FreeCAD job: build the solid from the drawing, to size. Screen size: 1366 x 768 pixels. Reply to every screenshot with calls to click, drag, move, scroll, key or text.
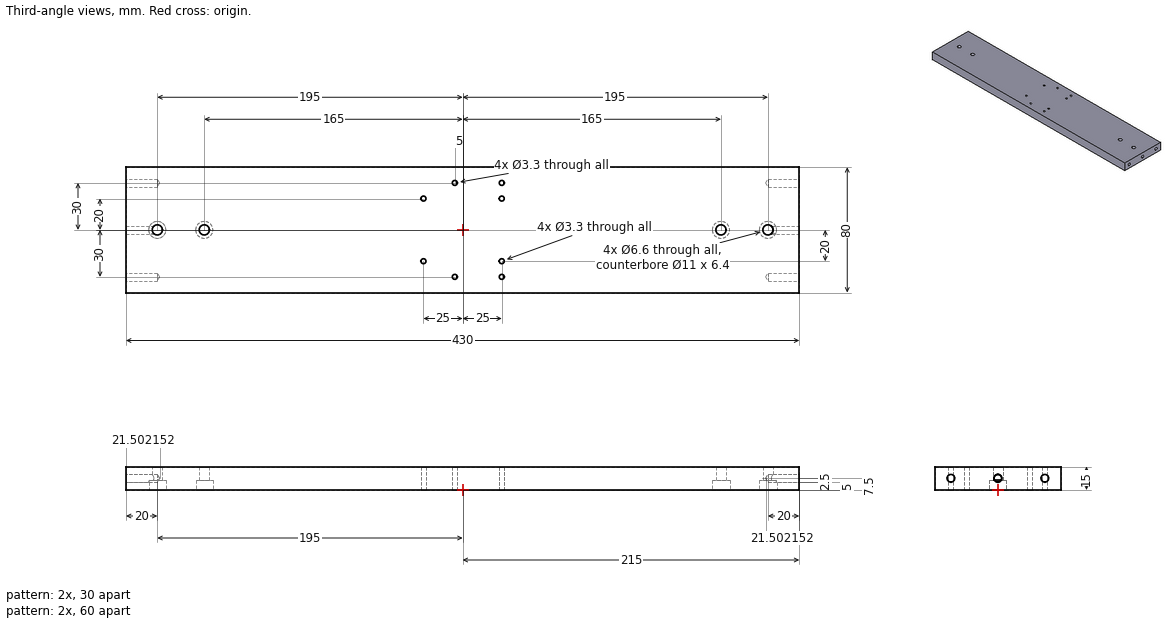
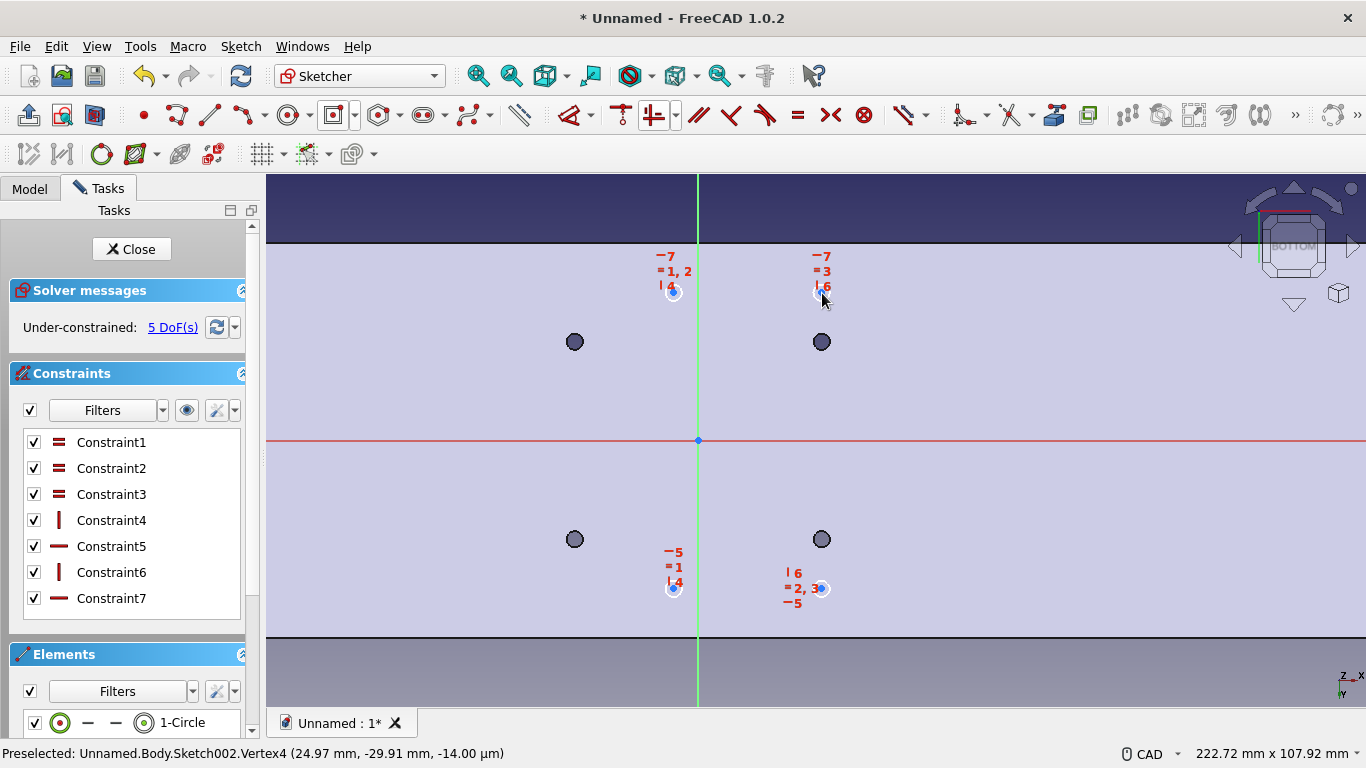
click(568, 116)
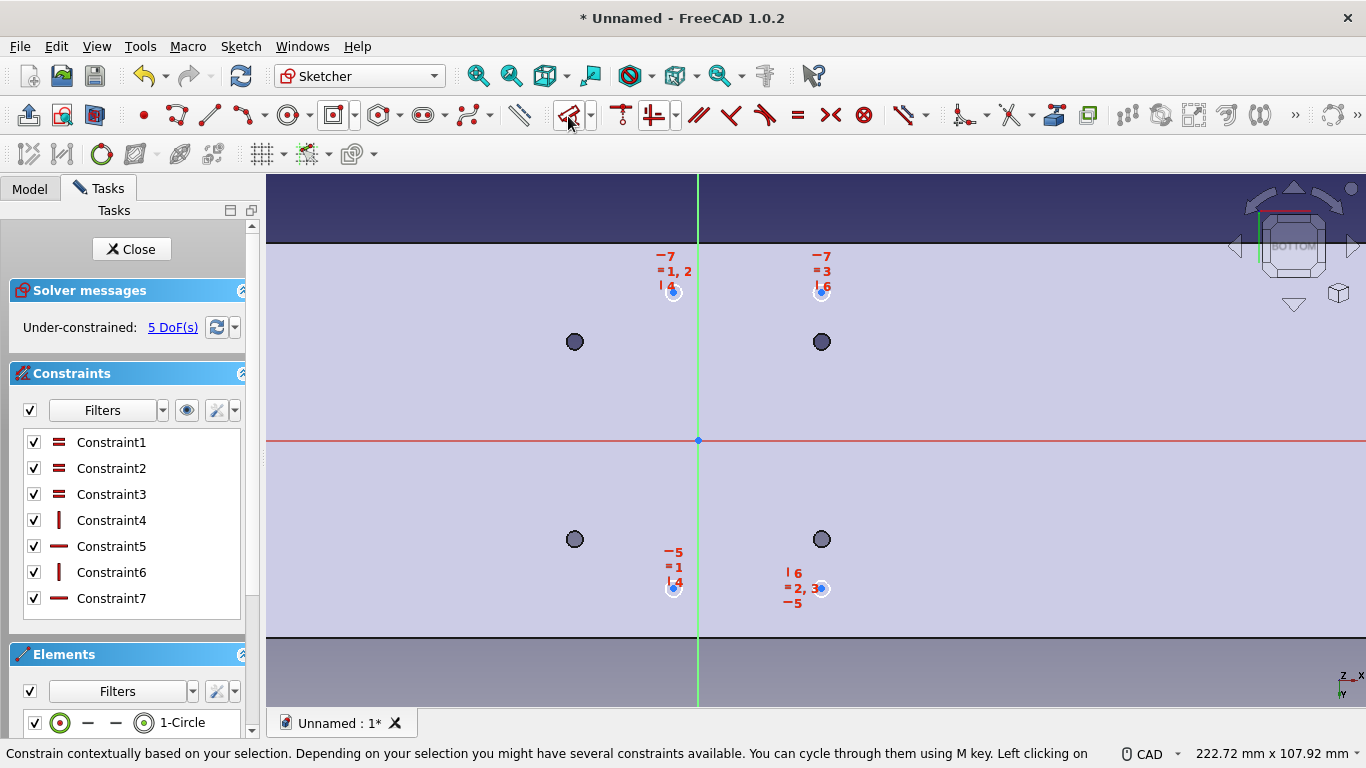
scroll(679, 583, up, 5)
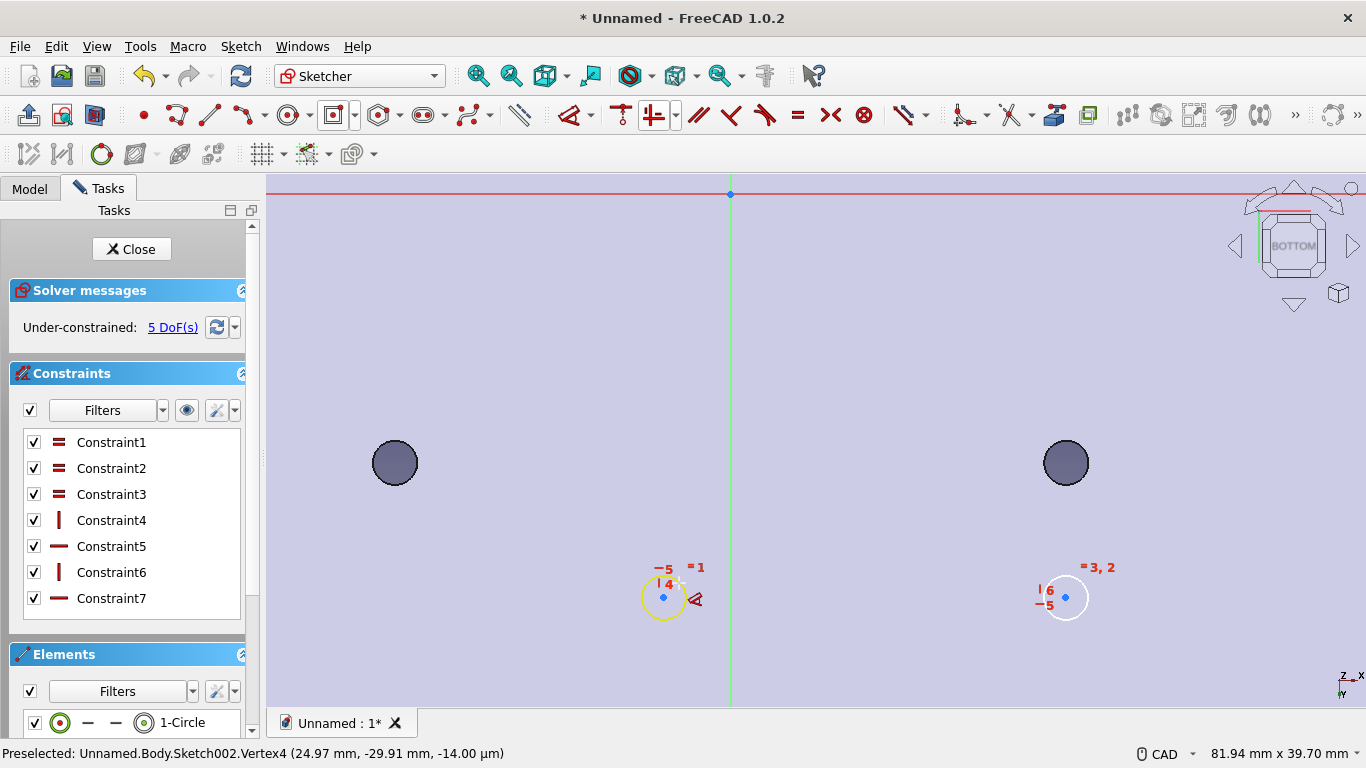
click(679, 582)
click(701, 559)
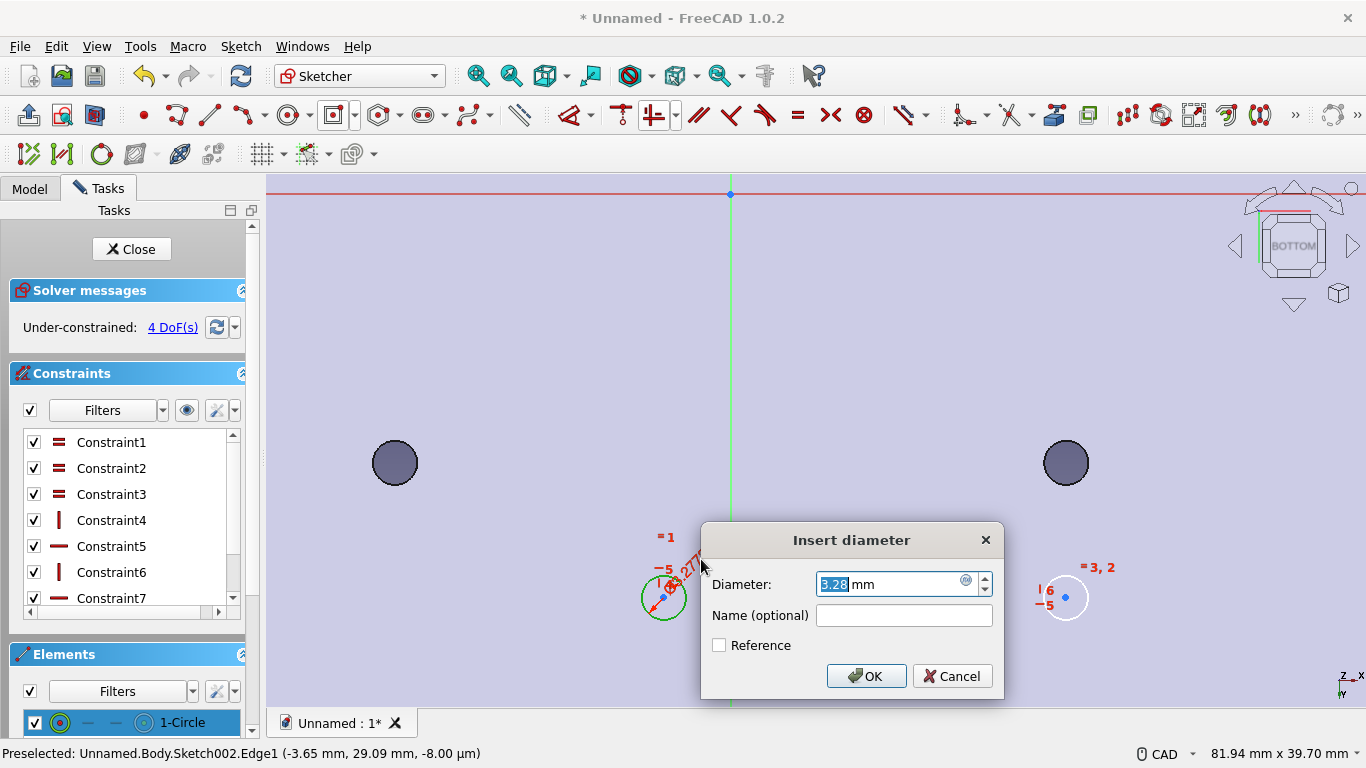
text(3.3)
key(Return)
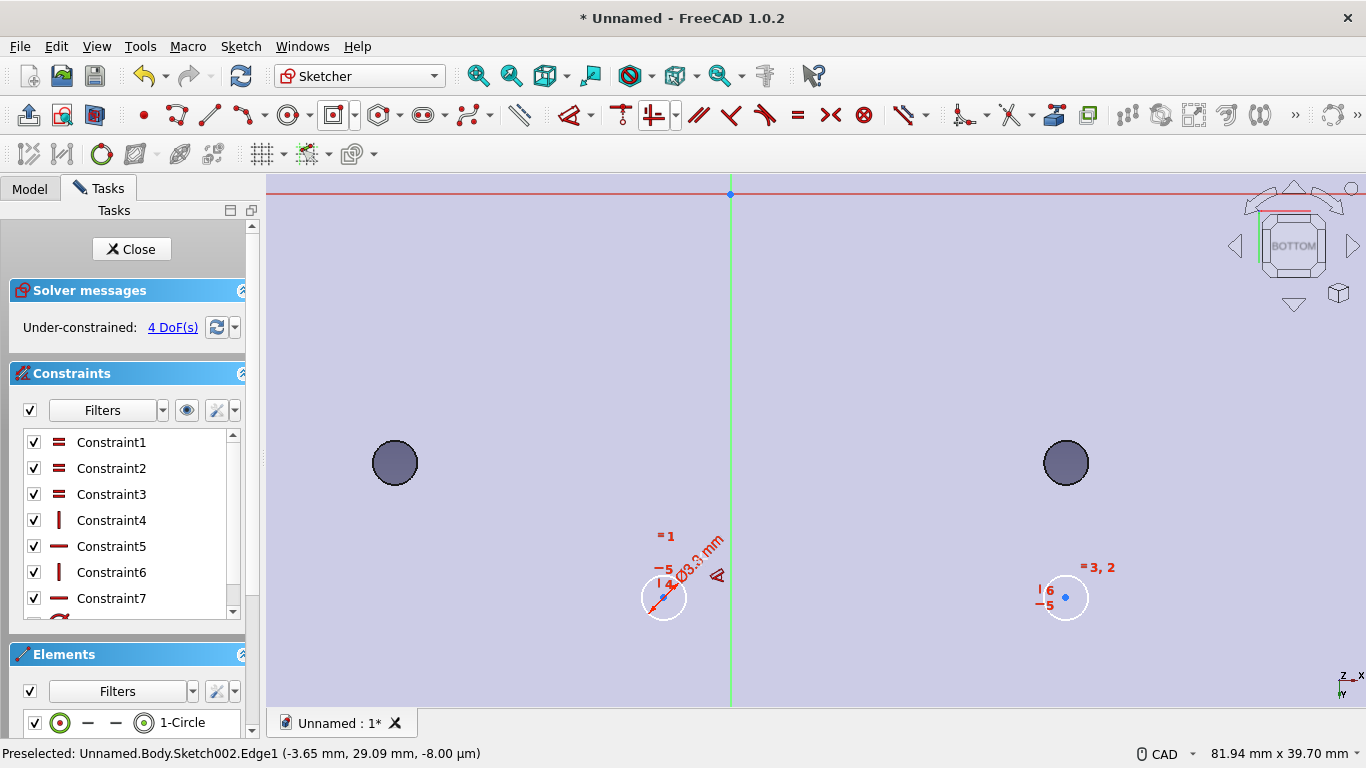
click(664, 598)
click(697, 632)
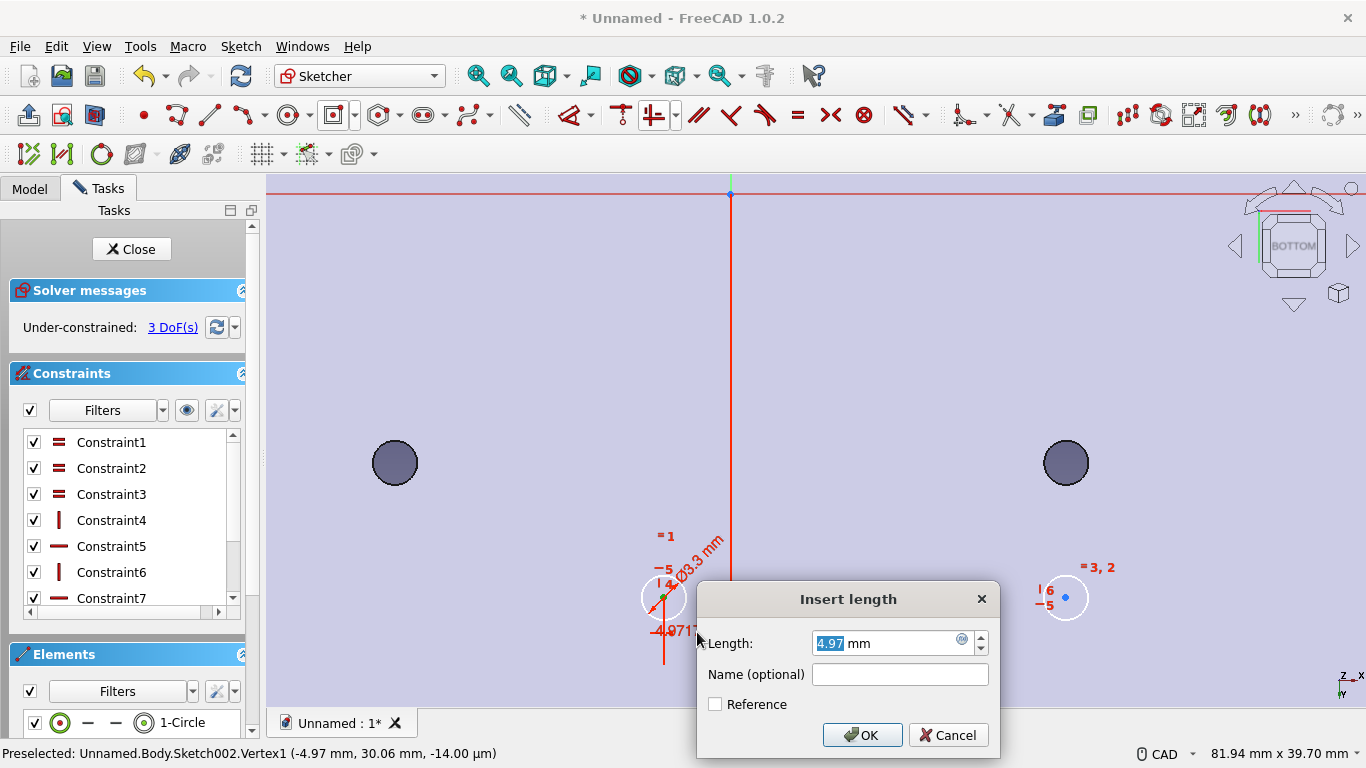
text(5)
key(Return)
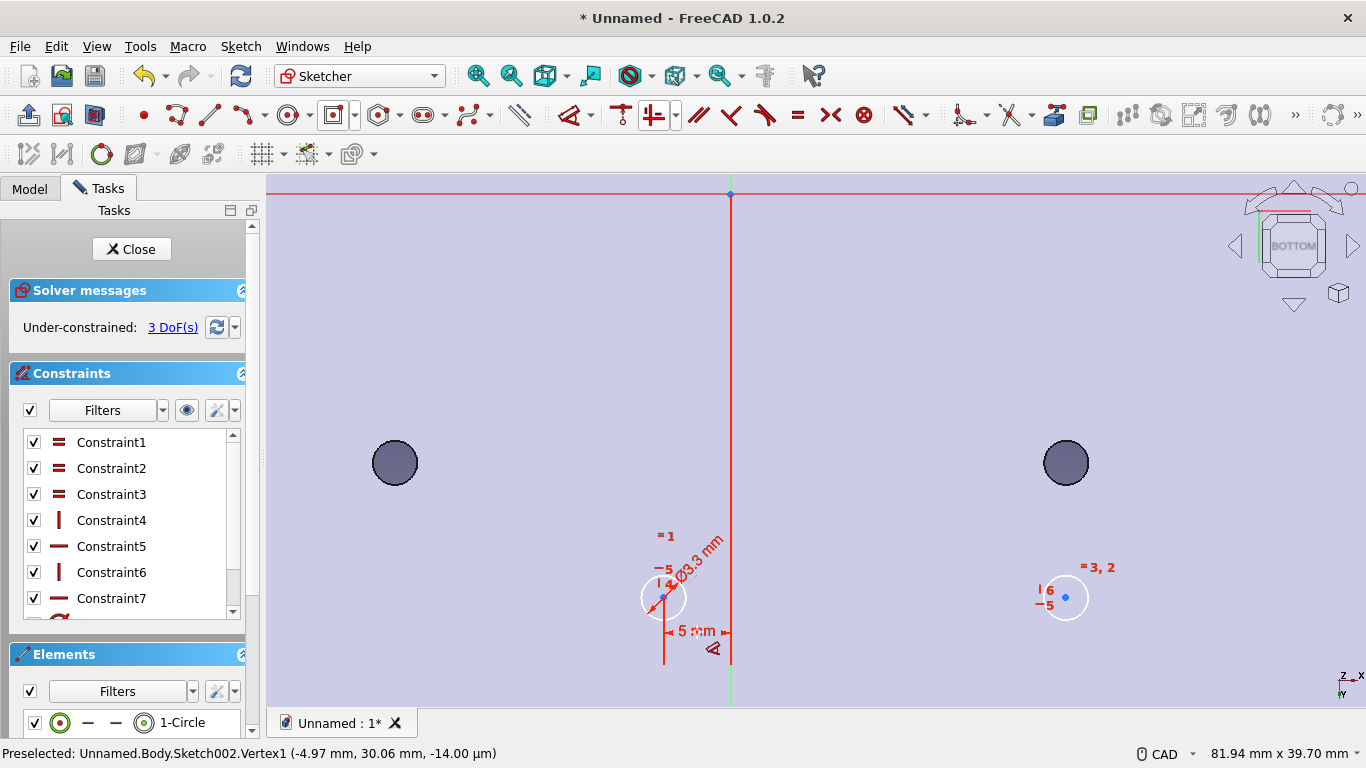
click(664, 598)
click(630, 400)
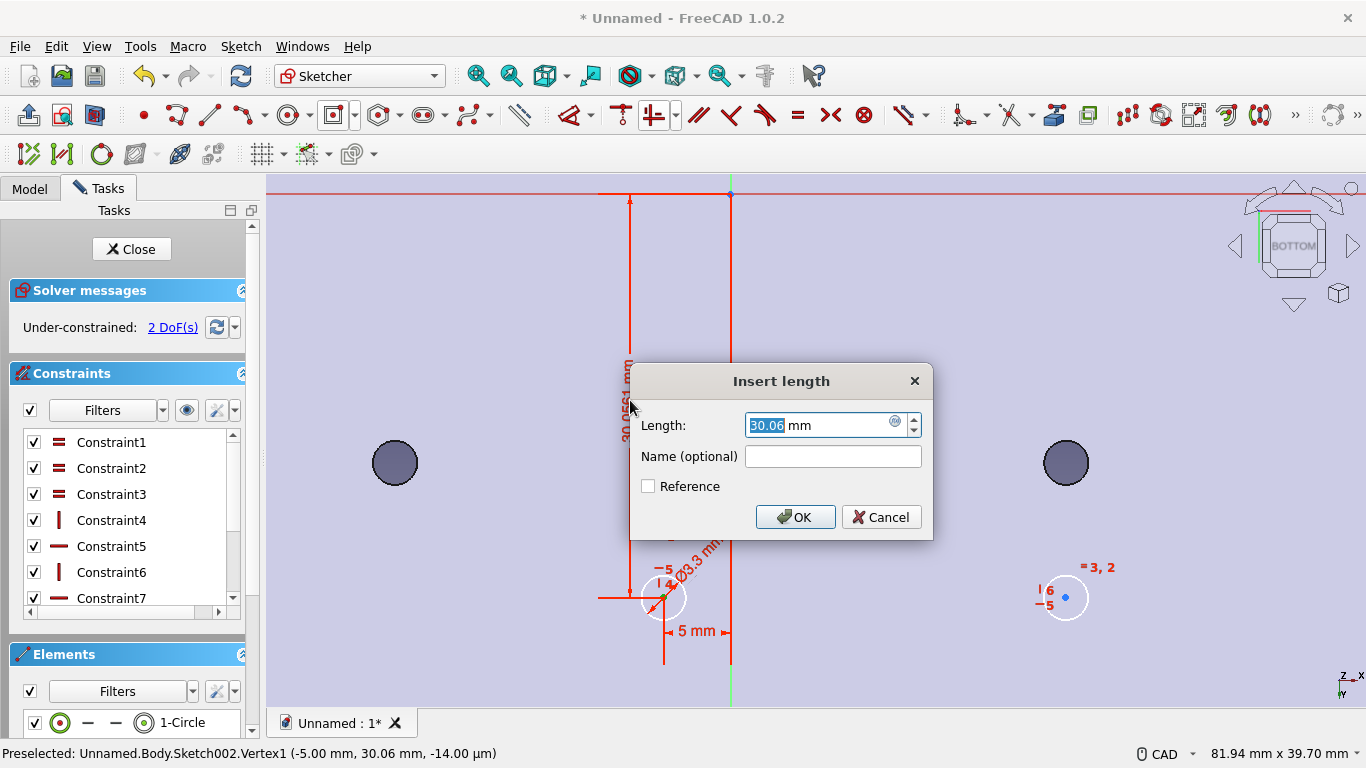
text(30)
key(Return)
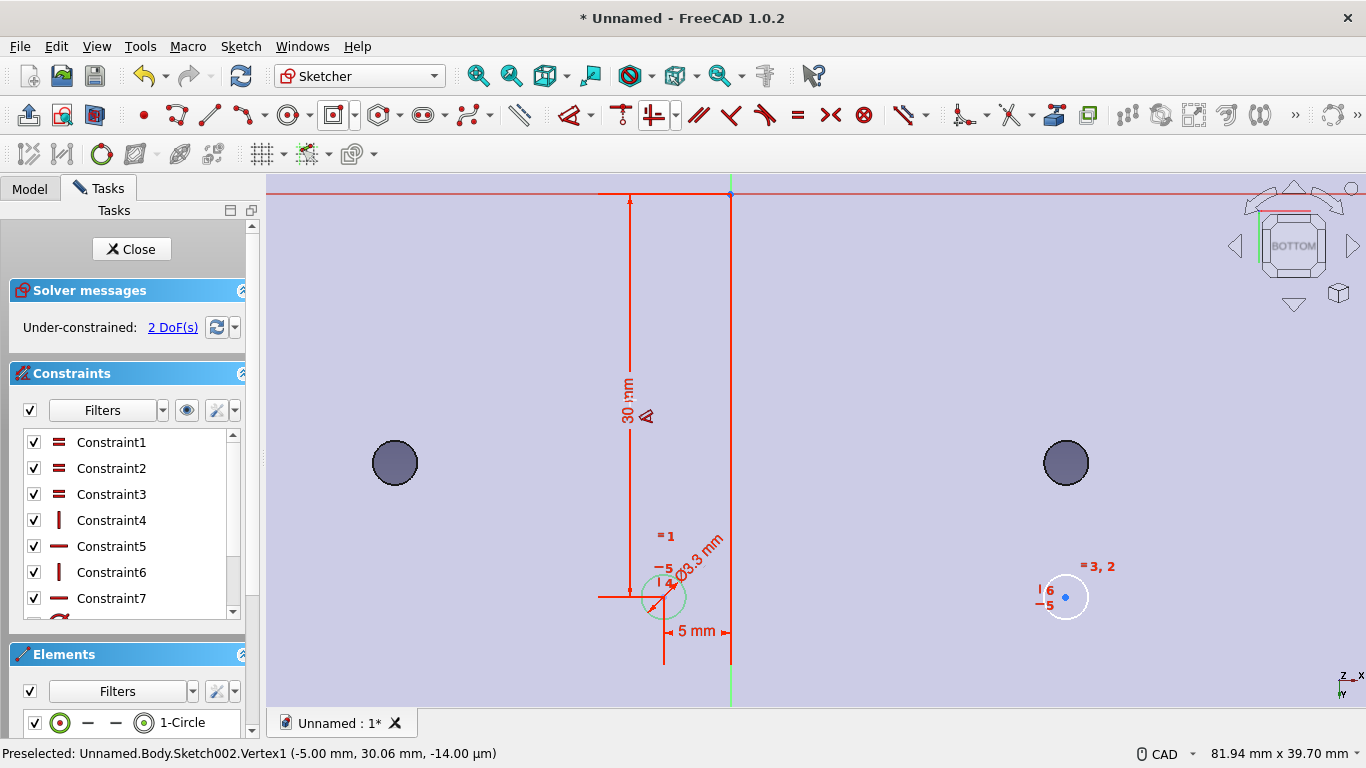
scroll(679, 584, down, 5)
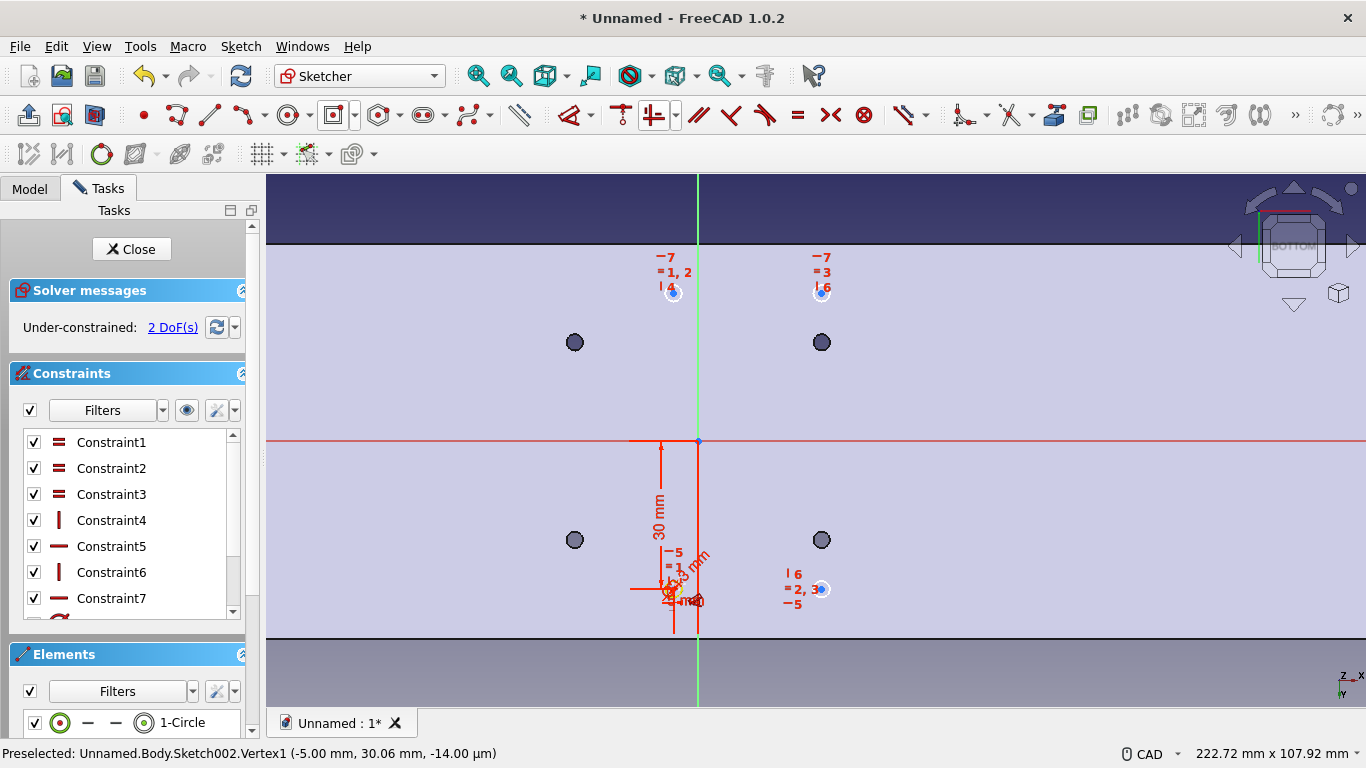
click(674, 293)
click(640, 367)